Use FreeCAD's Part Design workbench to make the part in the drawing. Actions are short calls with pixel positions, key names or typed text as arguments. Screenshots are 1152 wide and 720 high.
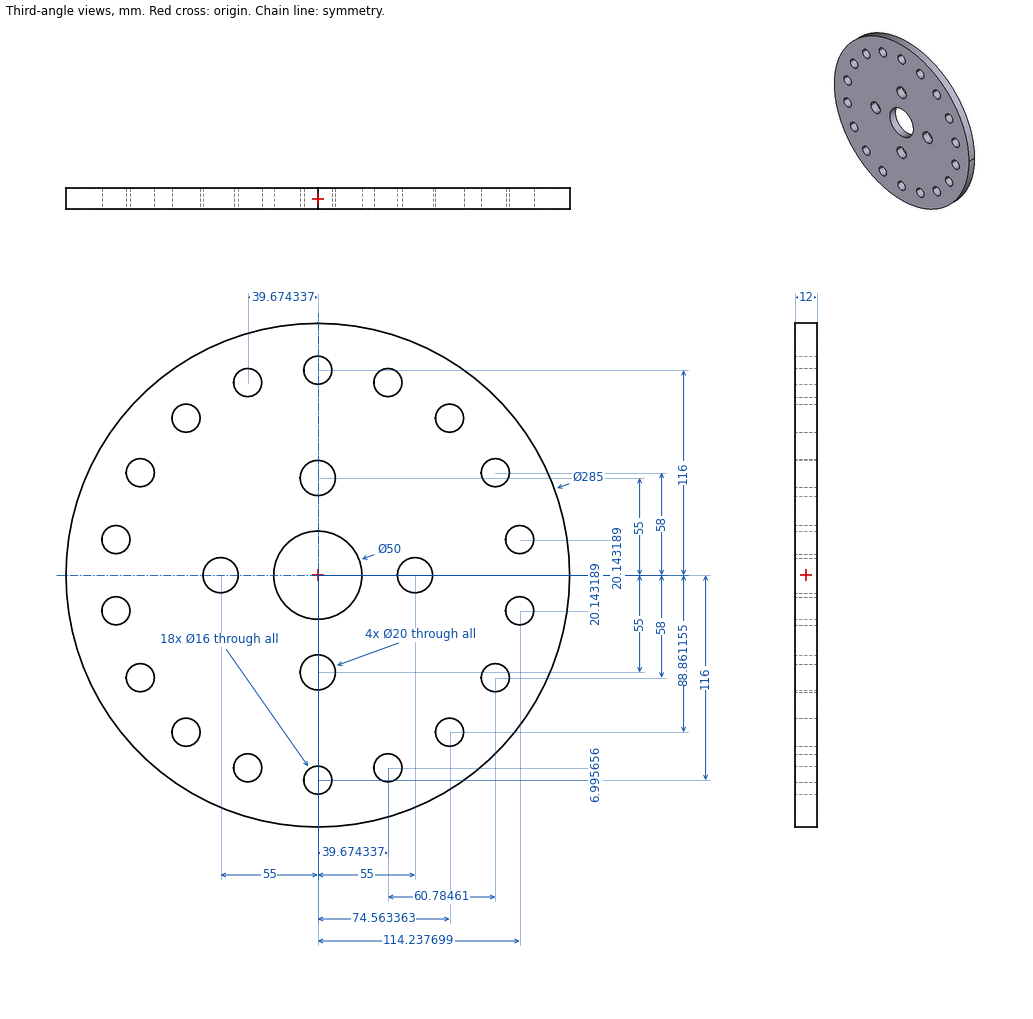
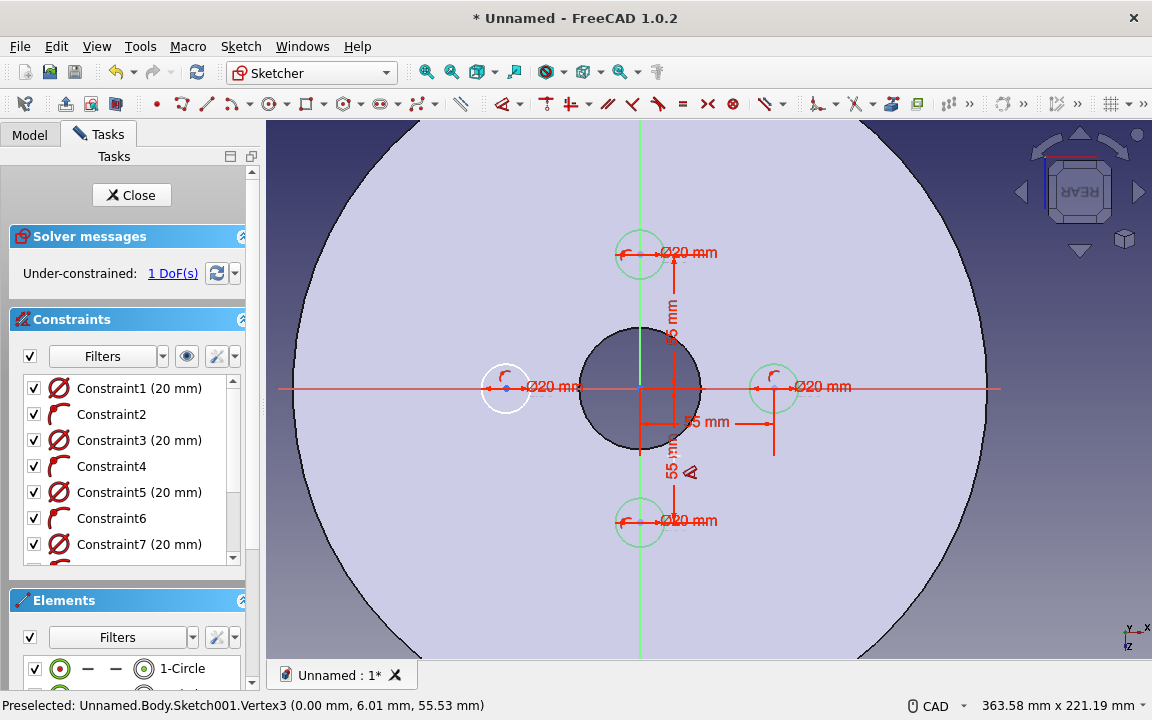
click(506, 389)
click(573, 423)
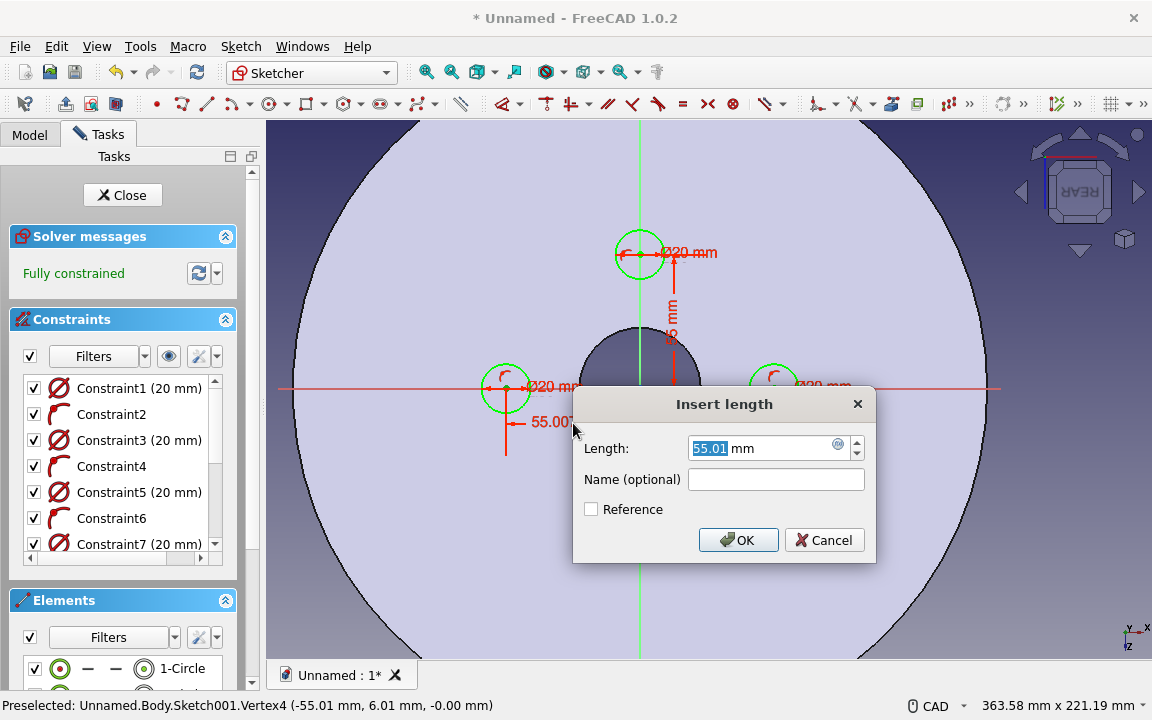
text(55)
key(Return)
key(Escape)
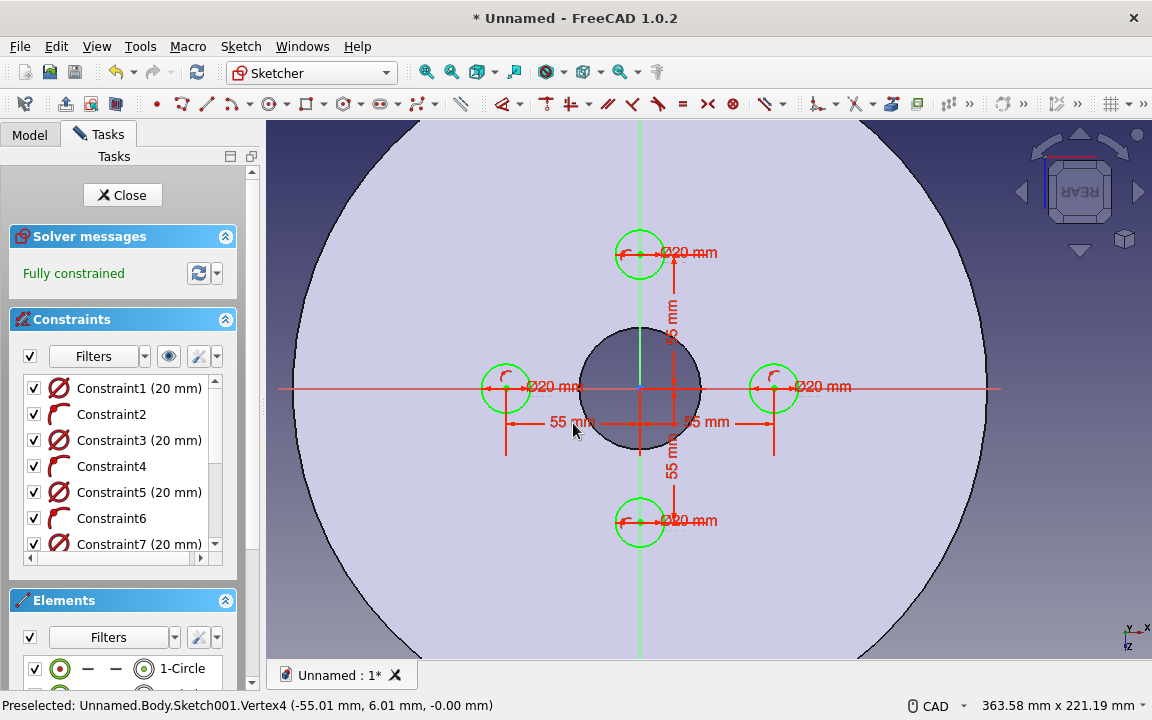
click(123, 195)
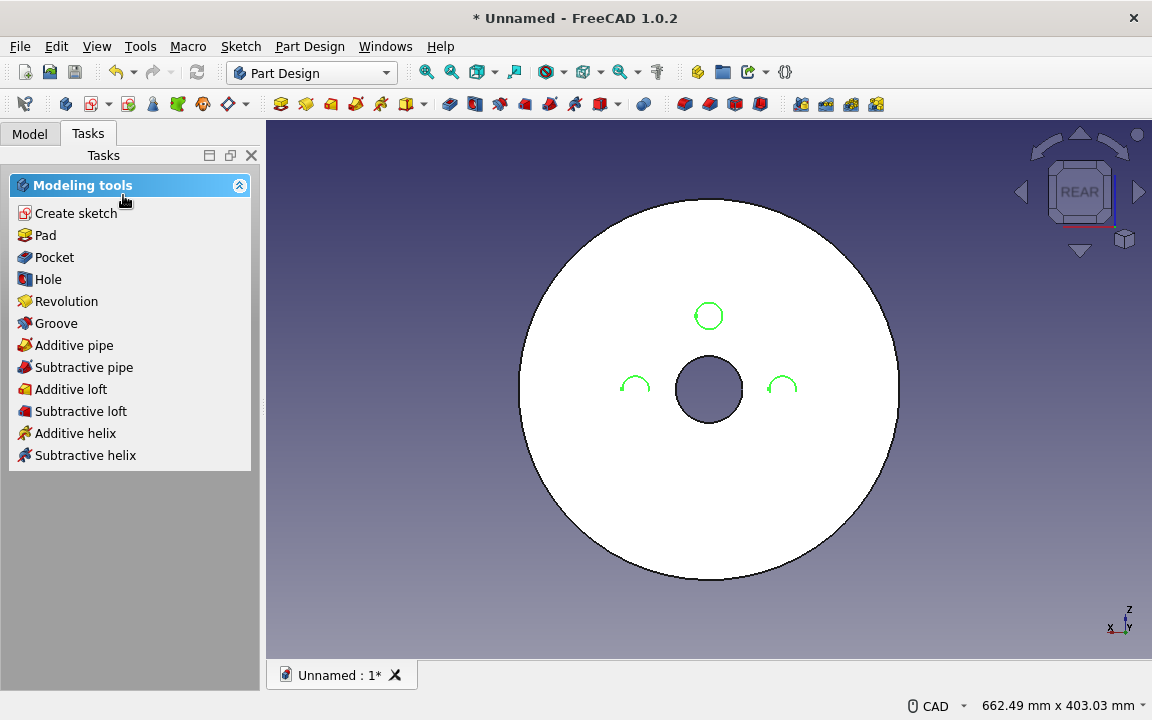
click(475, 104)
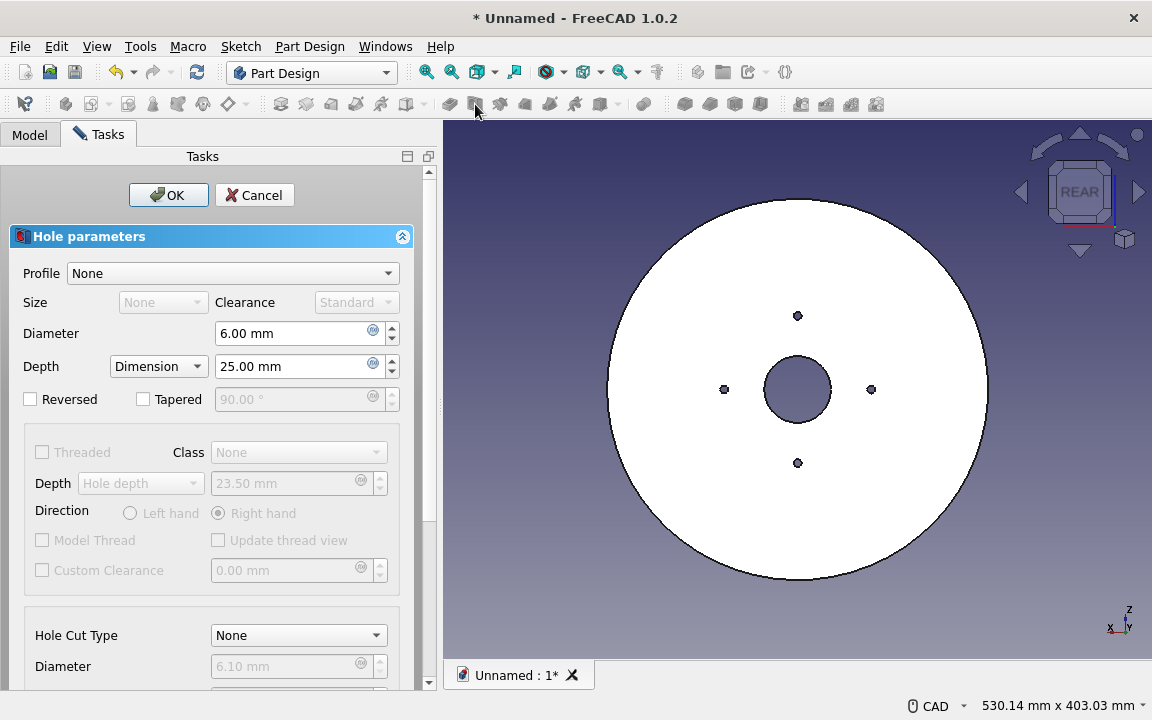
triple_click(300, 334)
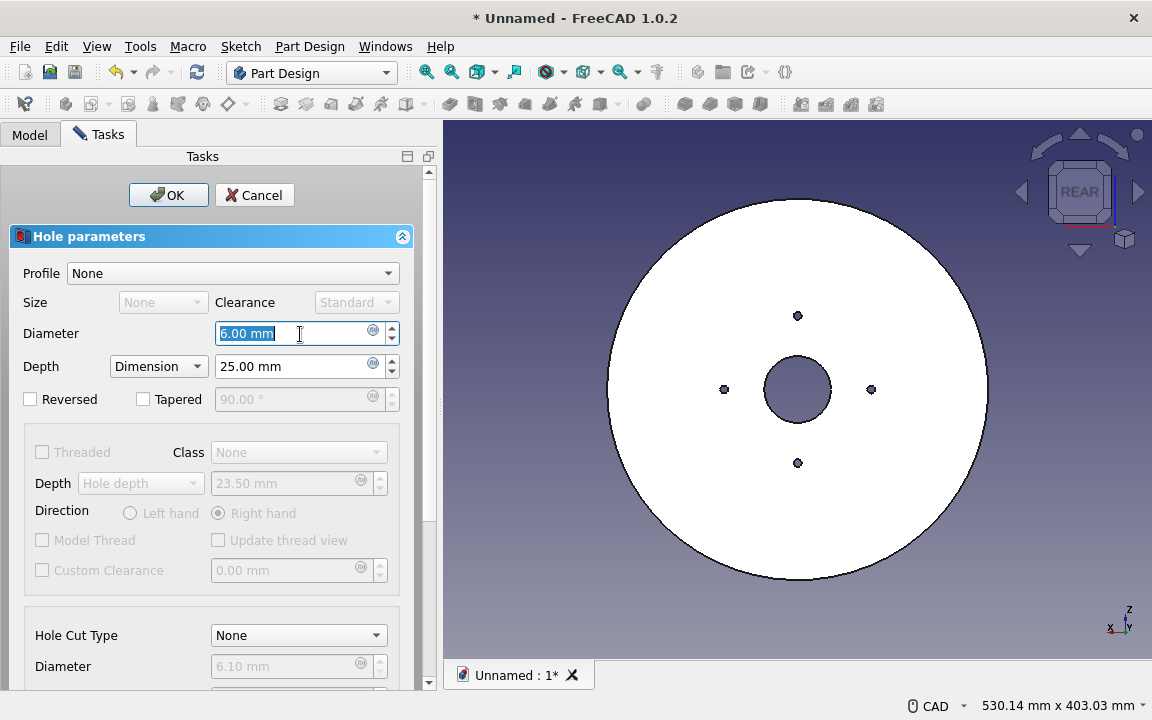
text(20)
key(Tab)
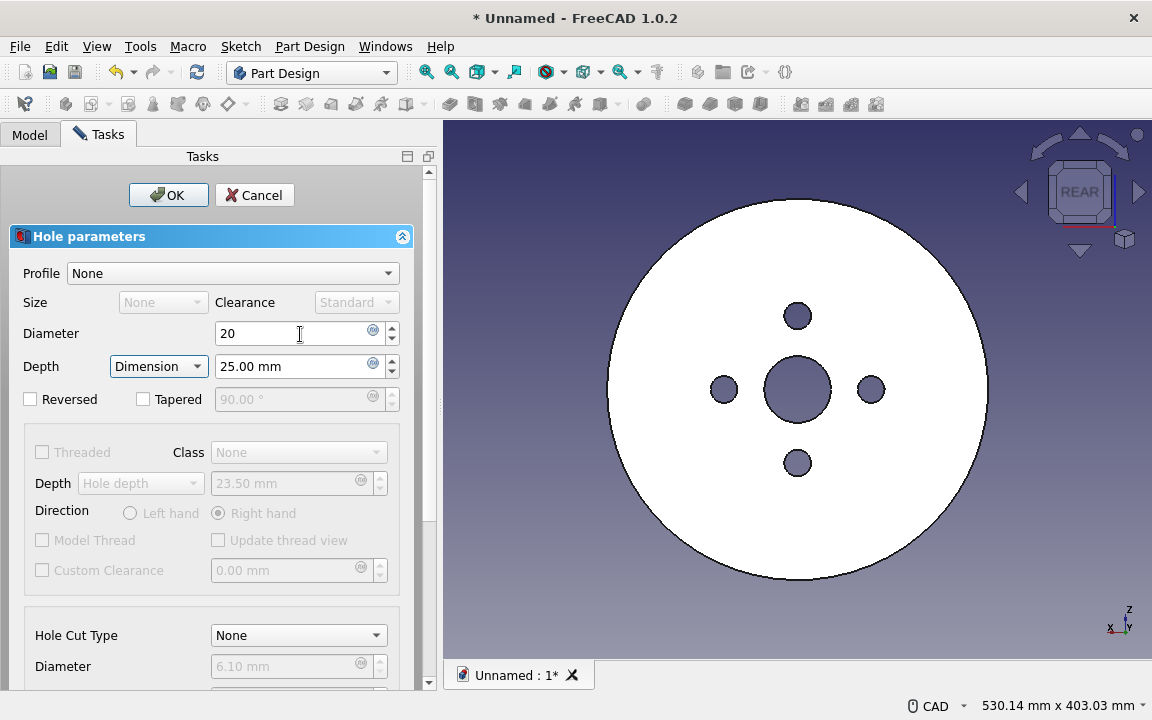
click(160, 366)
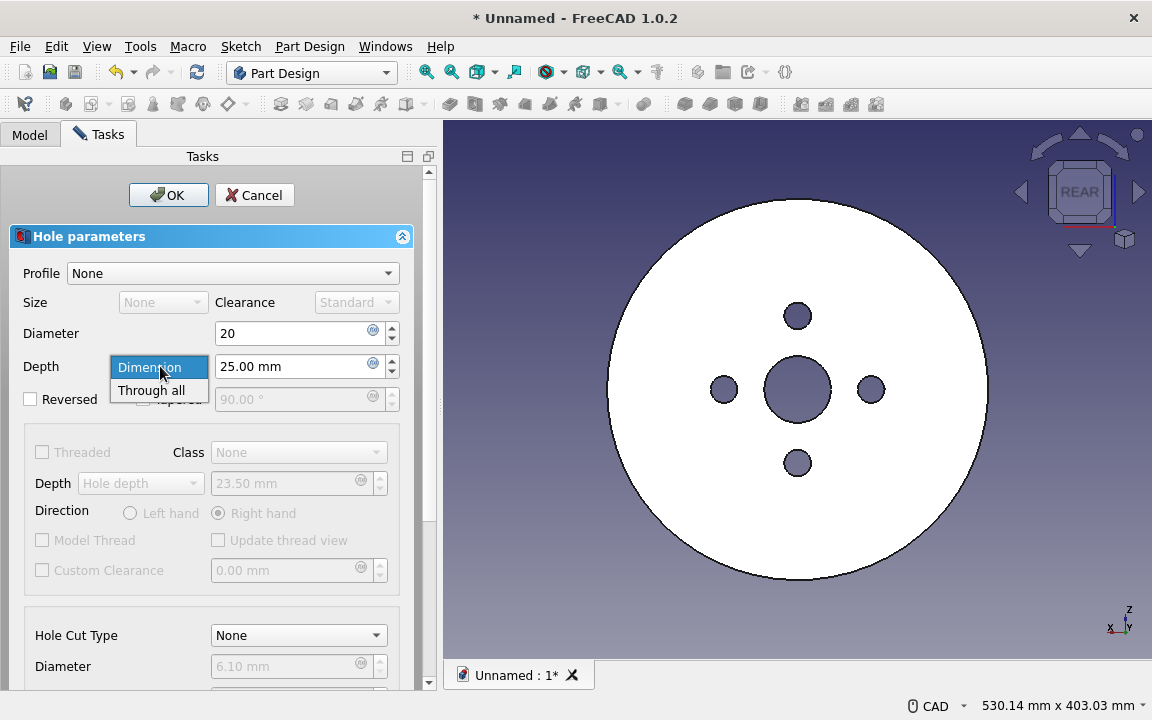
click(158, 390)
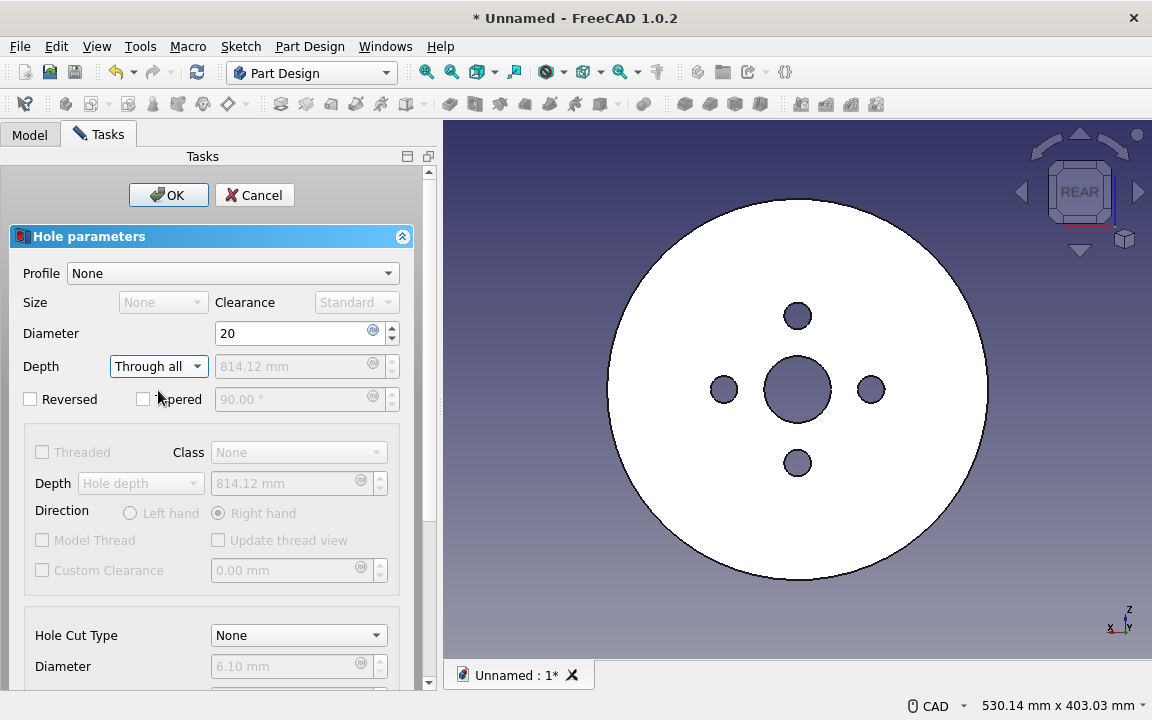
click(169, 195)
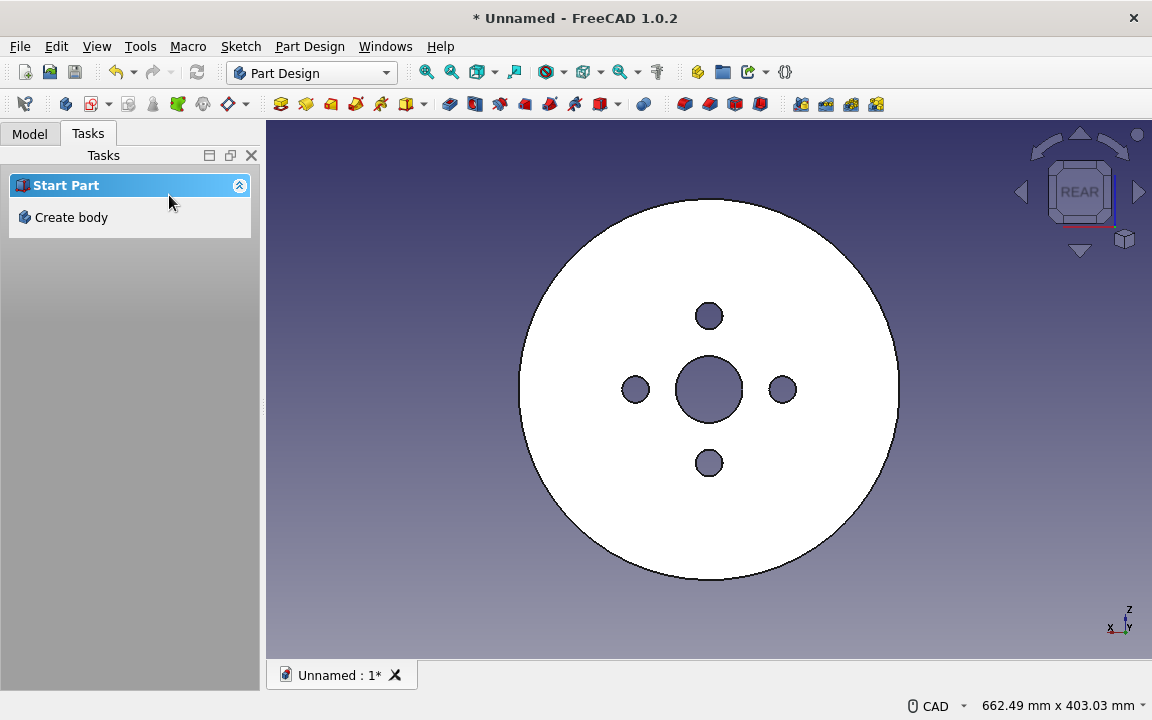
click(818, 334)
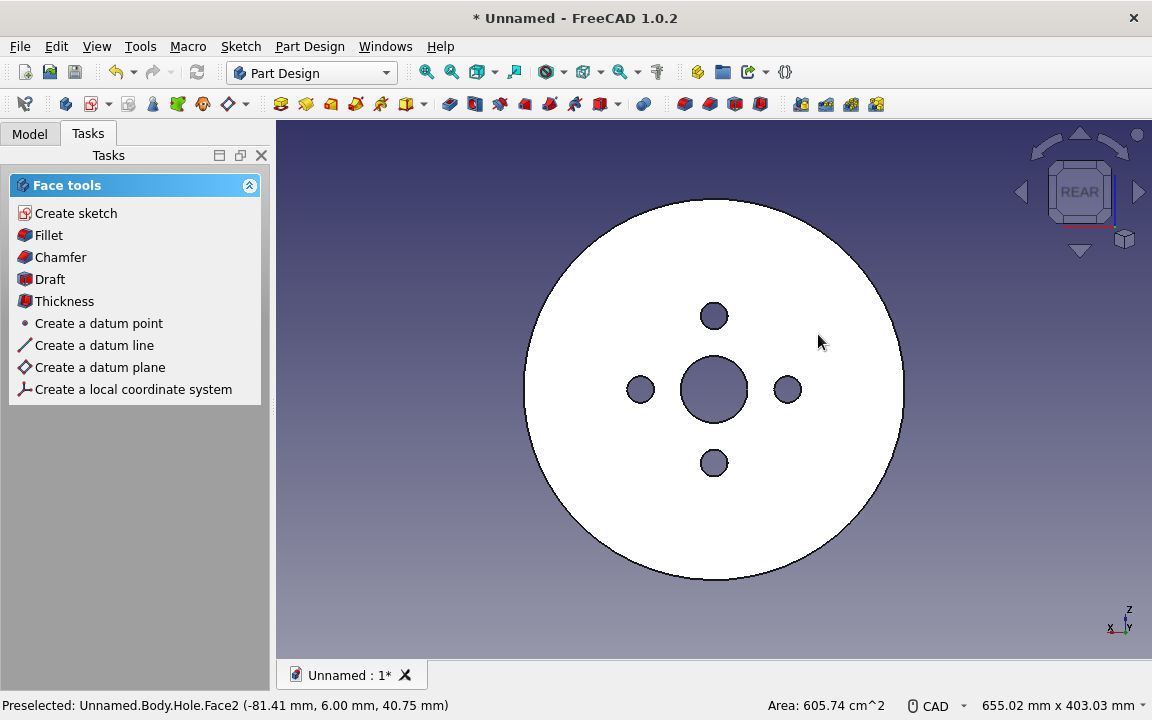
click(90, 104)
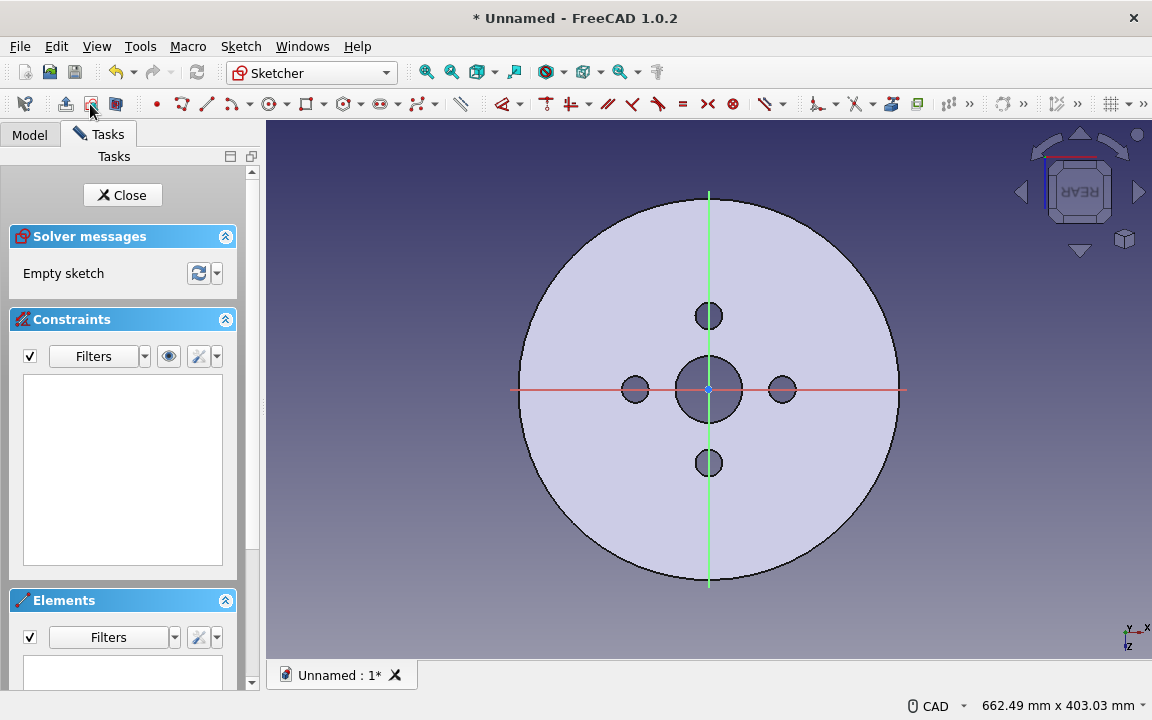
click(268, 104)